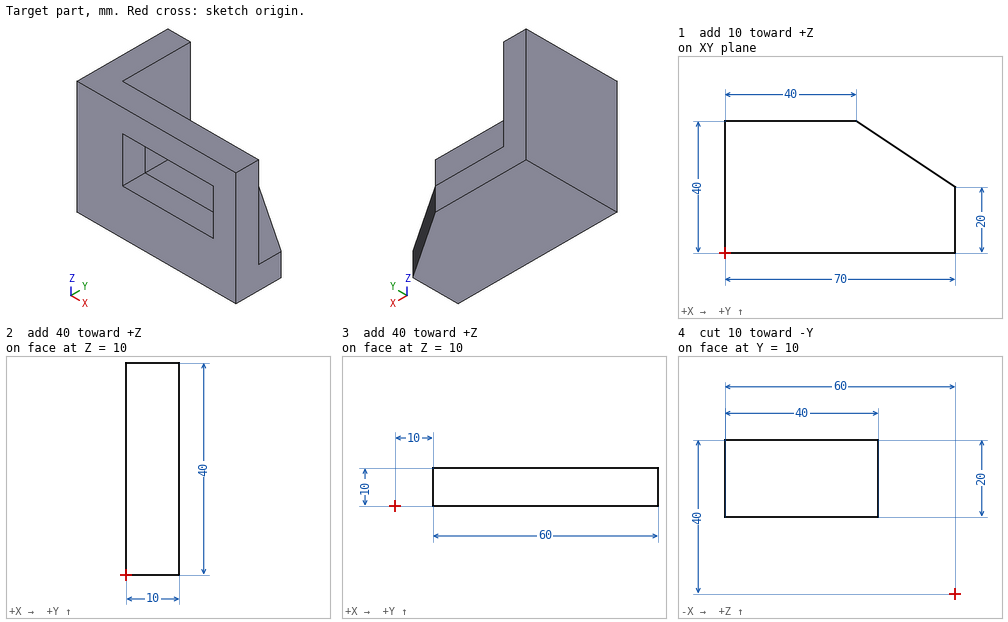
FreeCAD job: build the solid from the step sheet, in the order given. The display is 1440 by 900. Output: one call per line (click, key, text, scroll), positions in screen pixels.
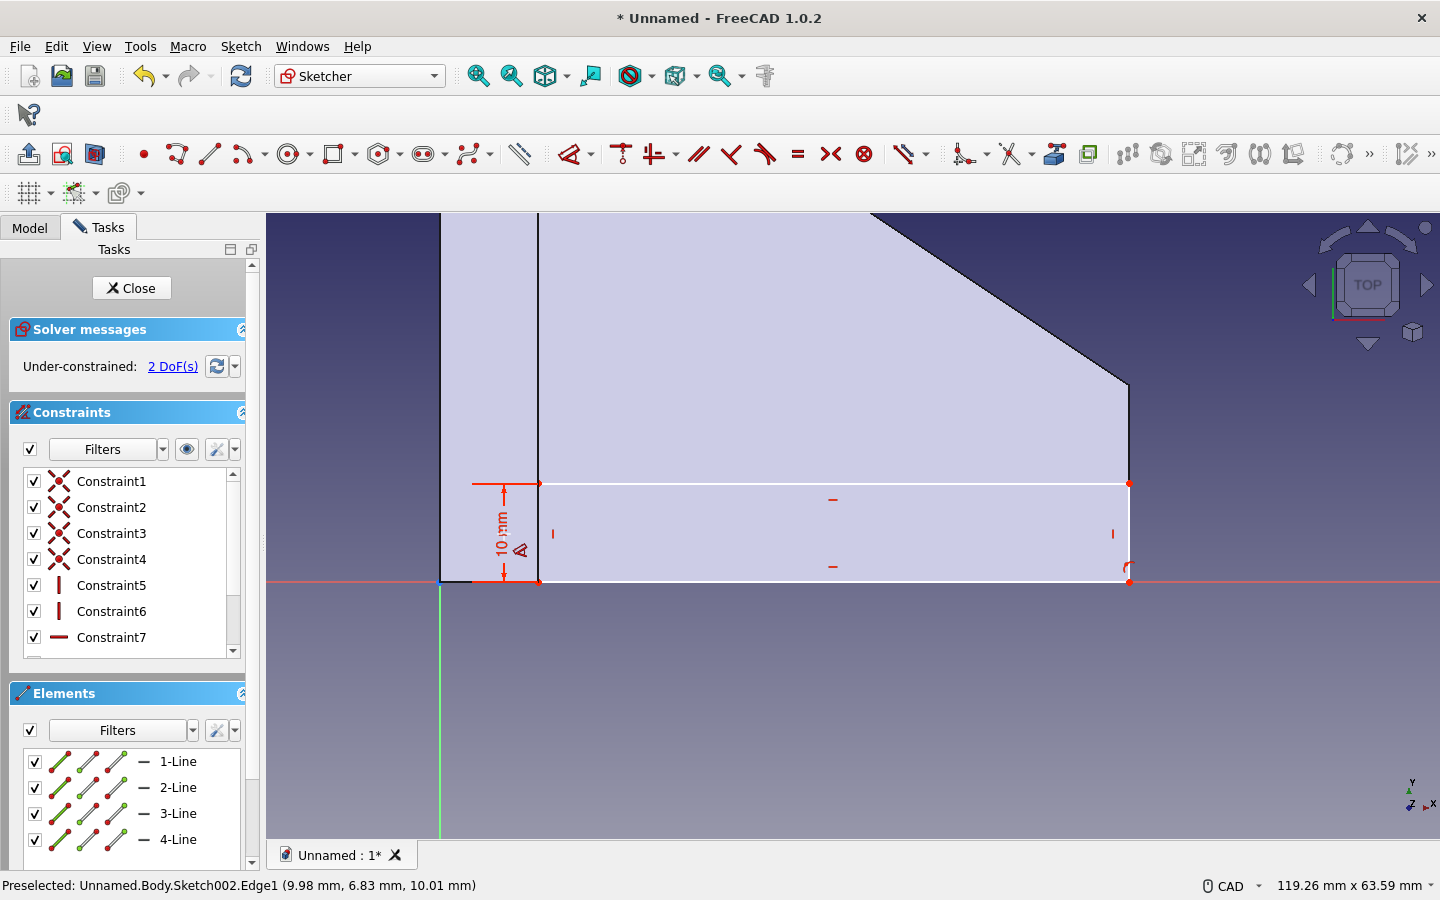
click(715, 582)
click(834, 616)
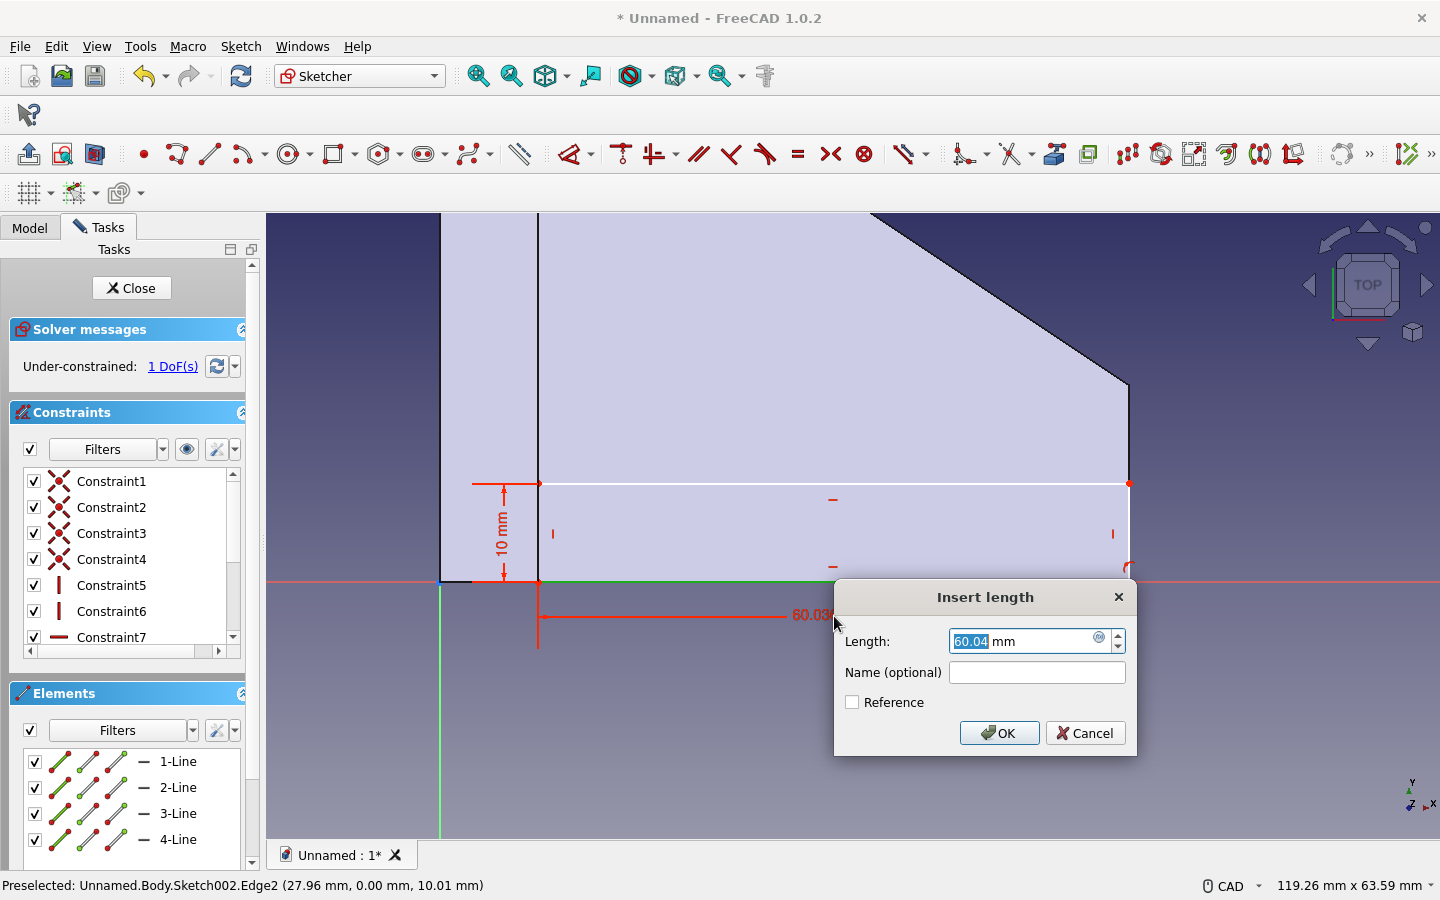
text(60)
key(Return)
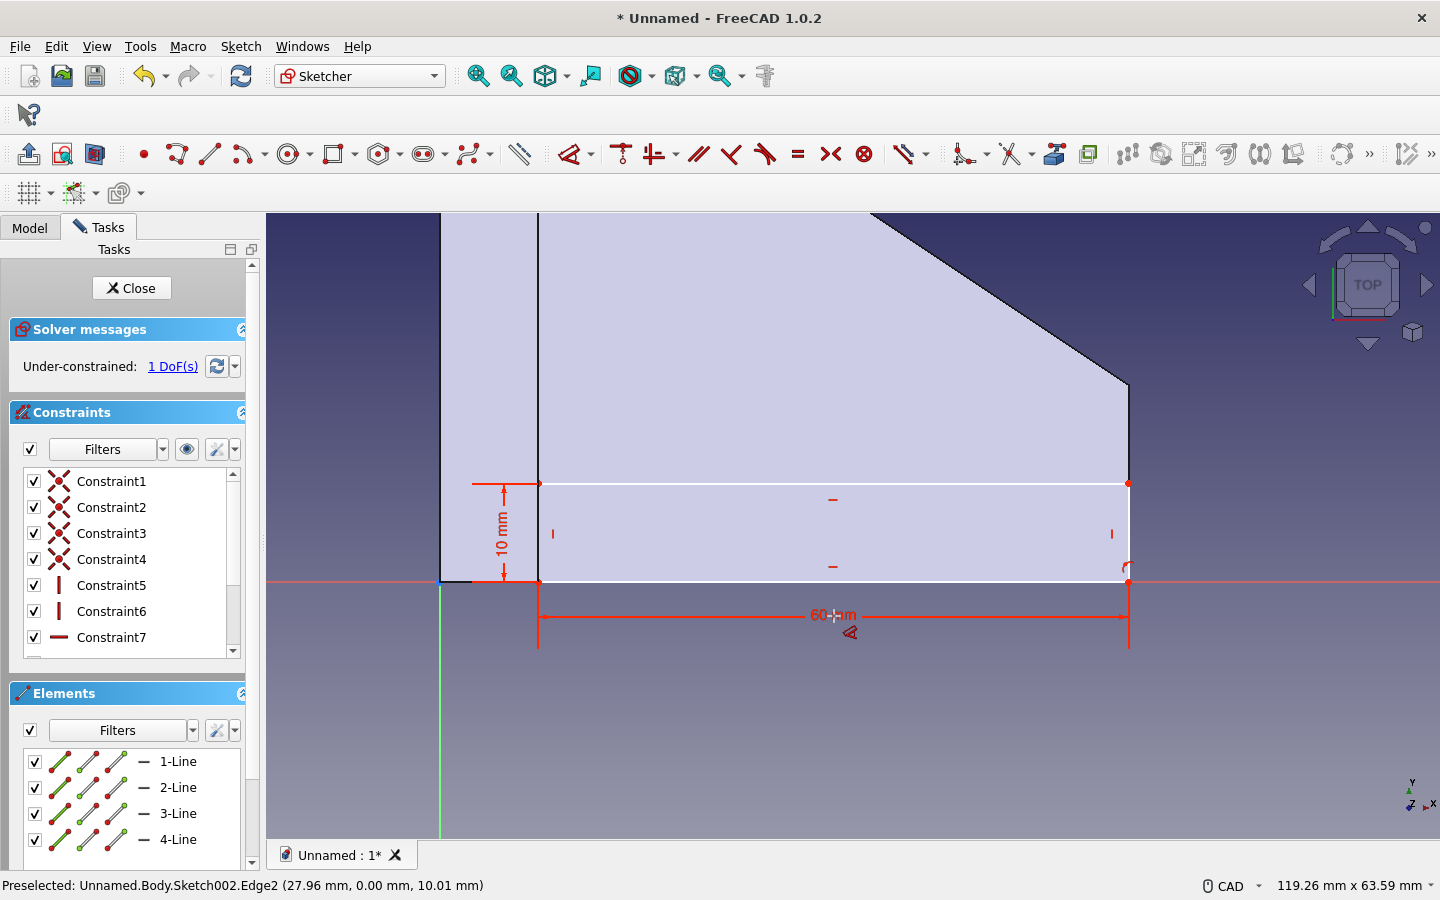
click(538, 484)
click(489, 450)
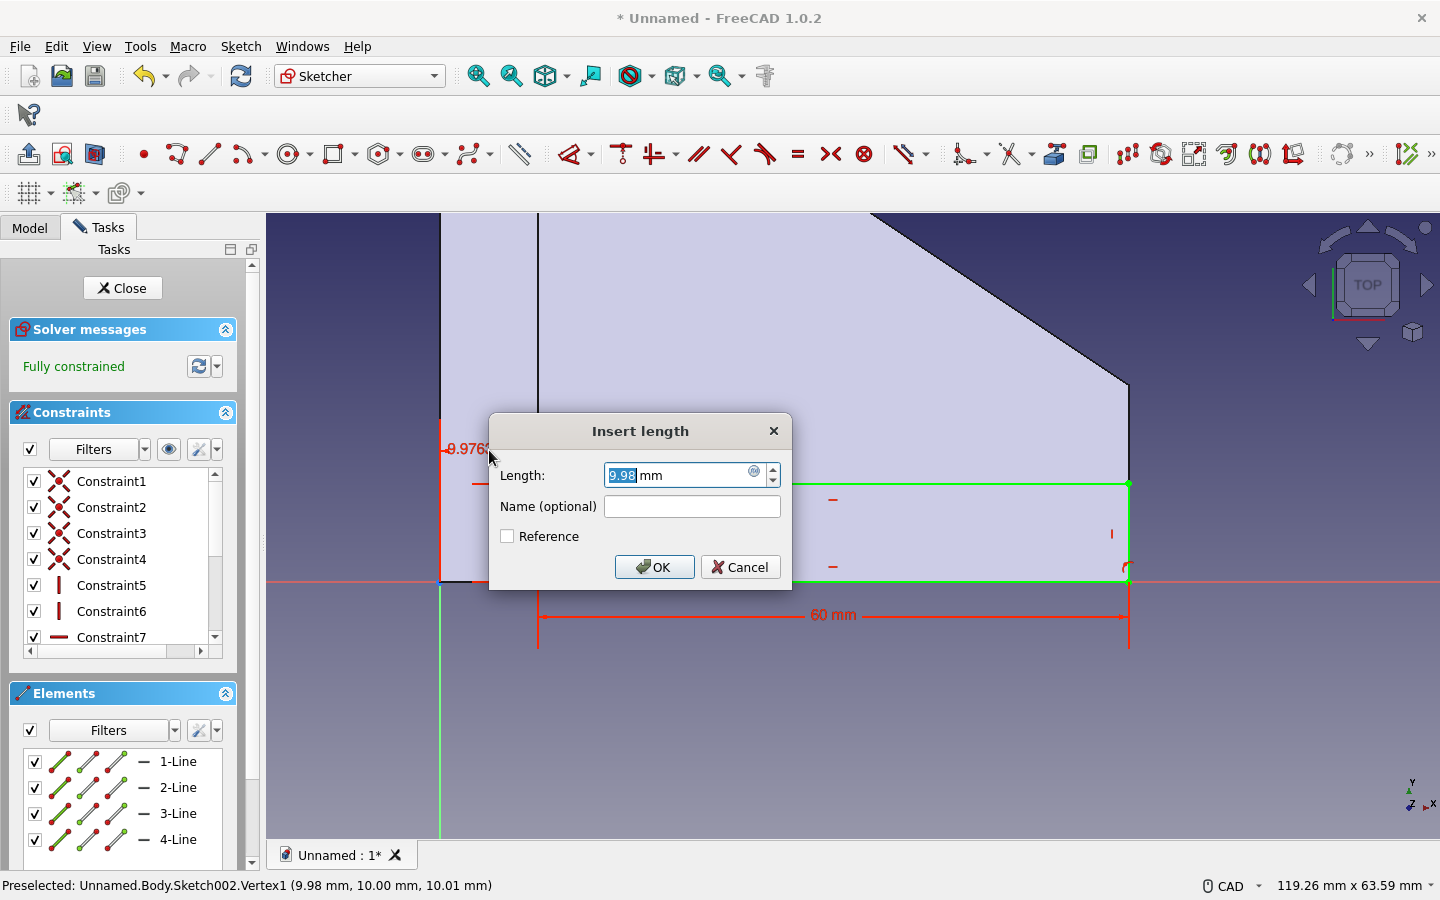
text(10)
key(Return)
key(Escape)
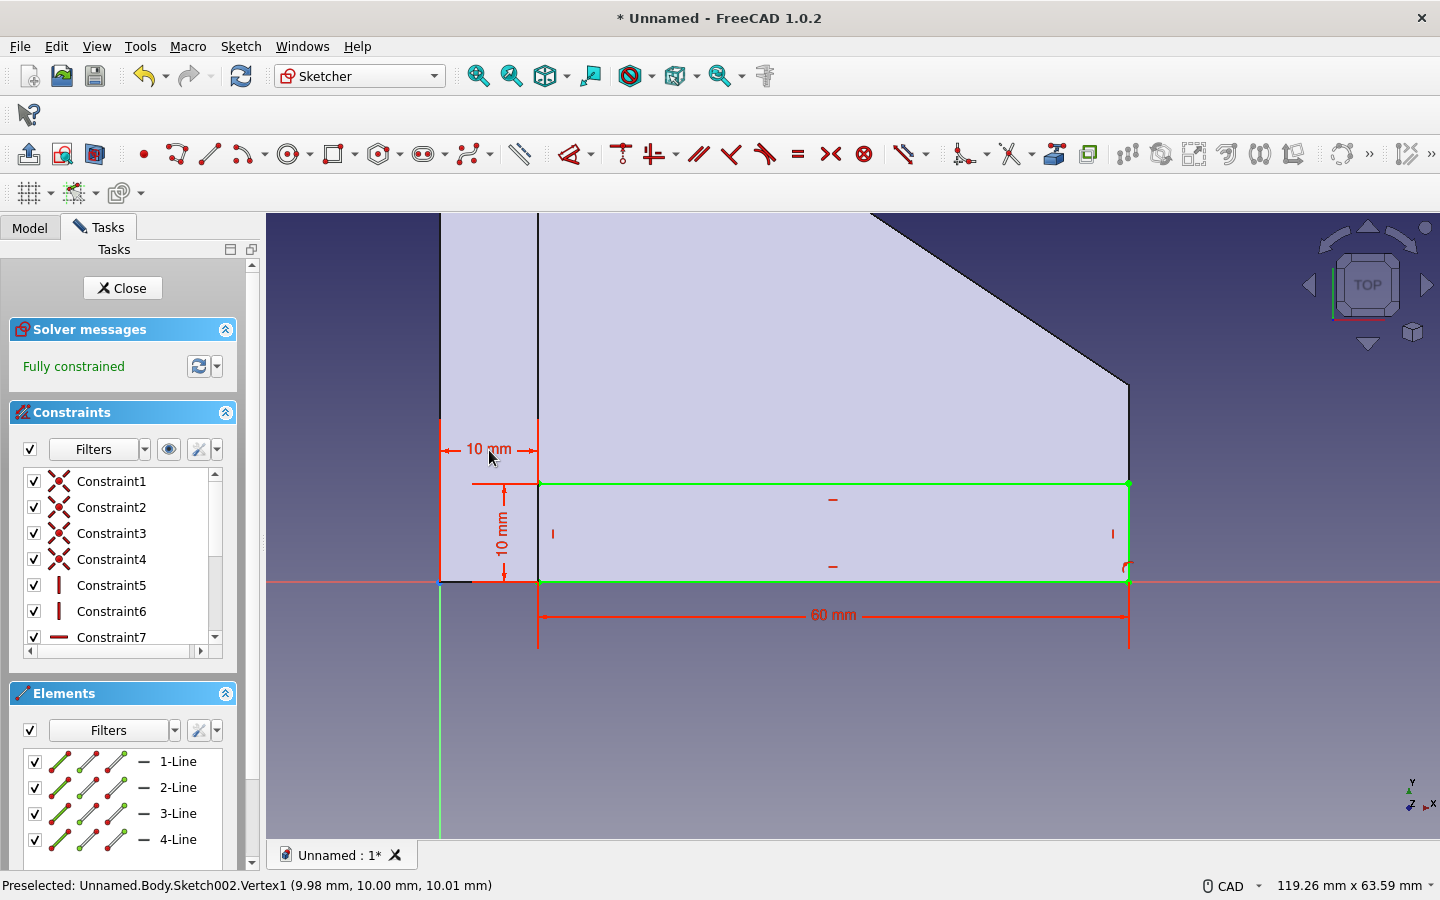
click(123, 288)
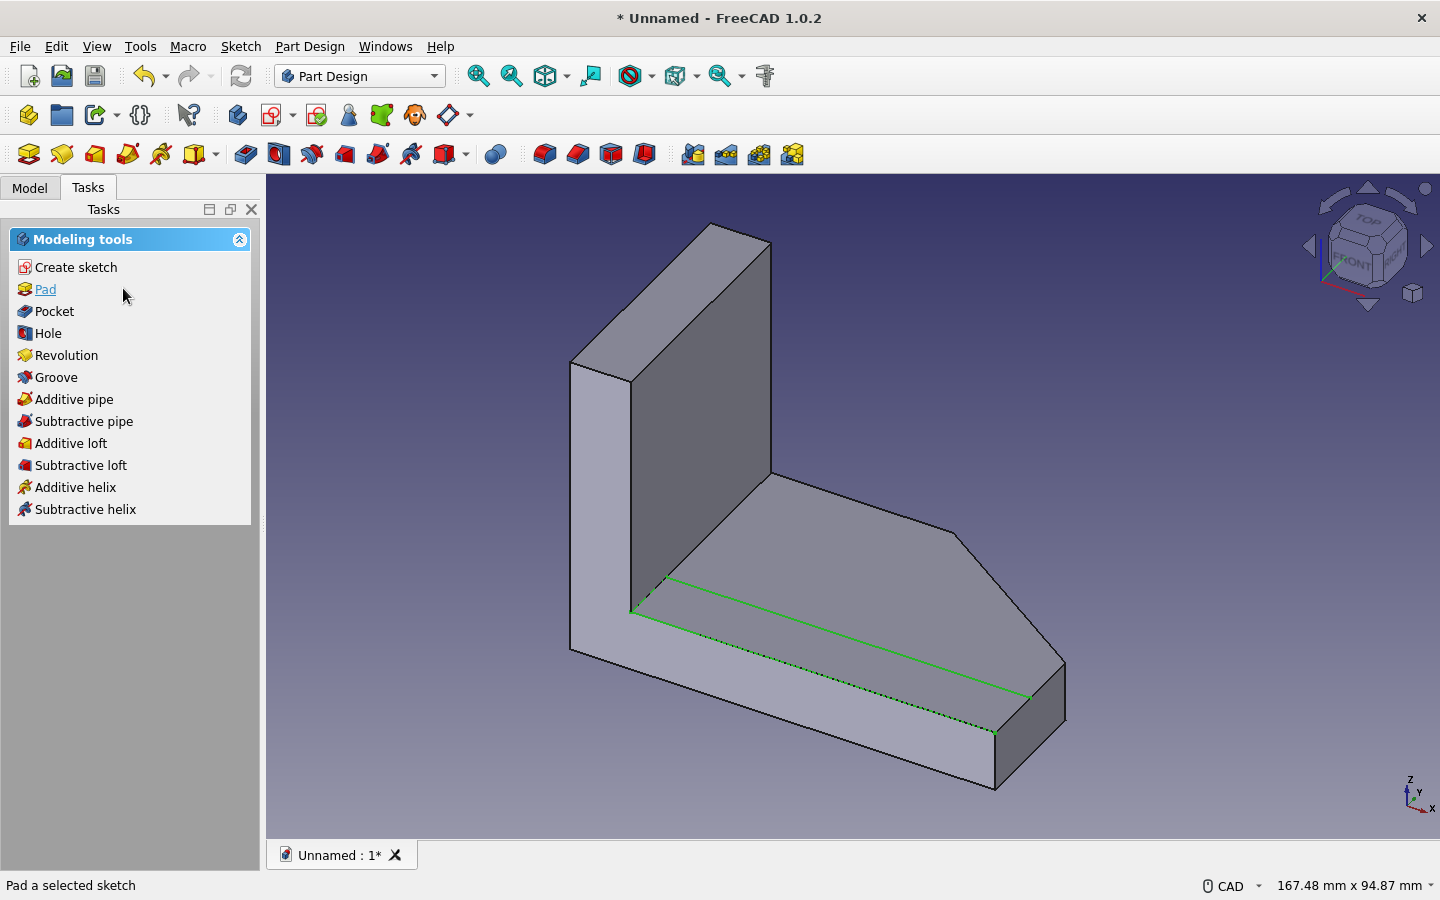
click(29, 154)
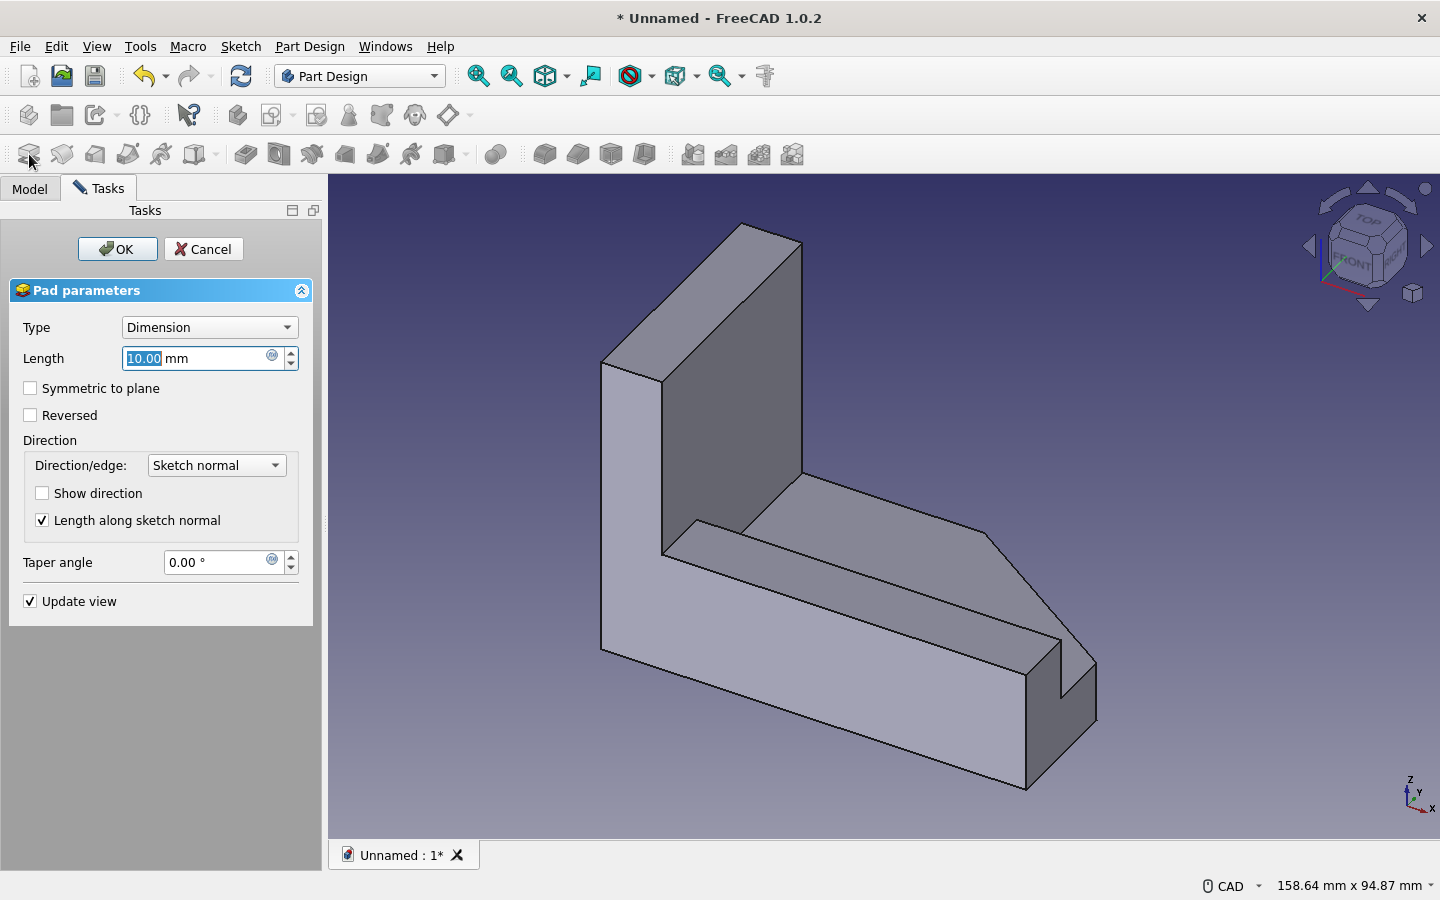
text(40)
key(Tab)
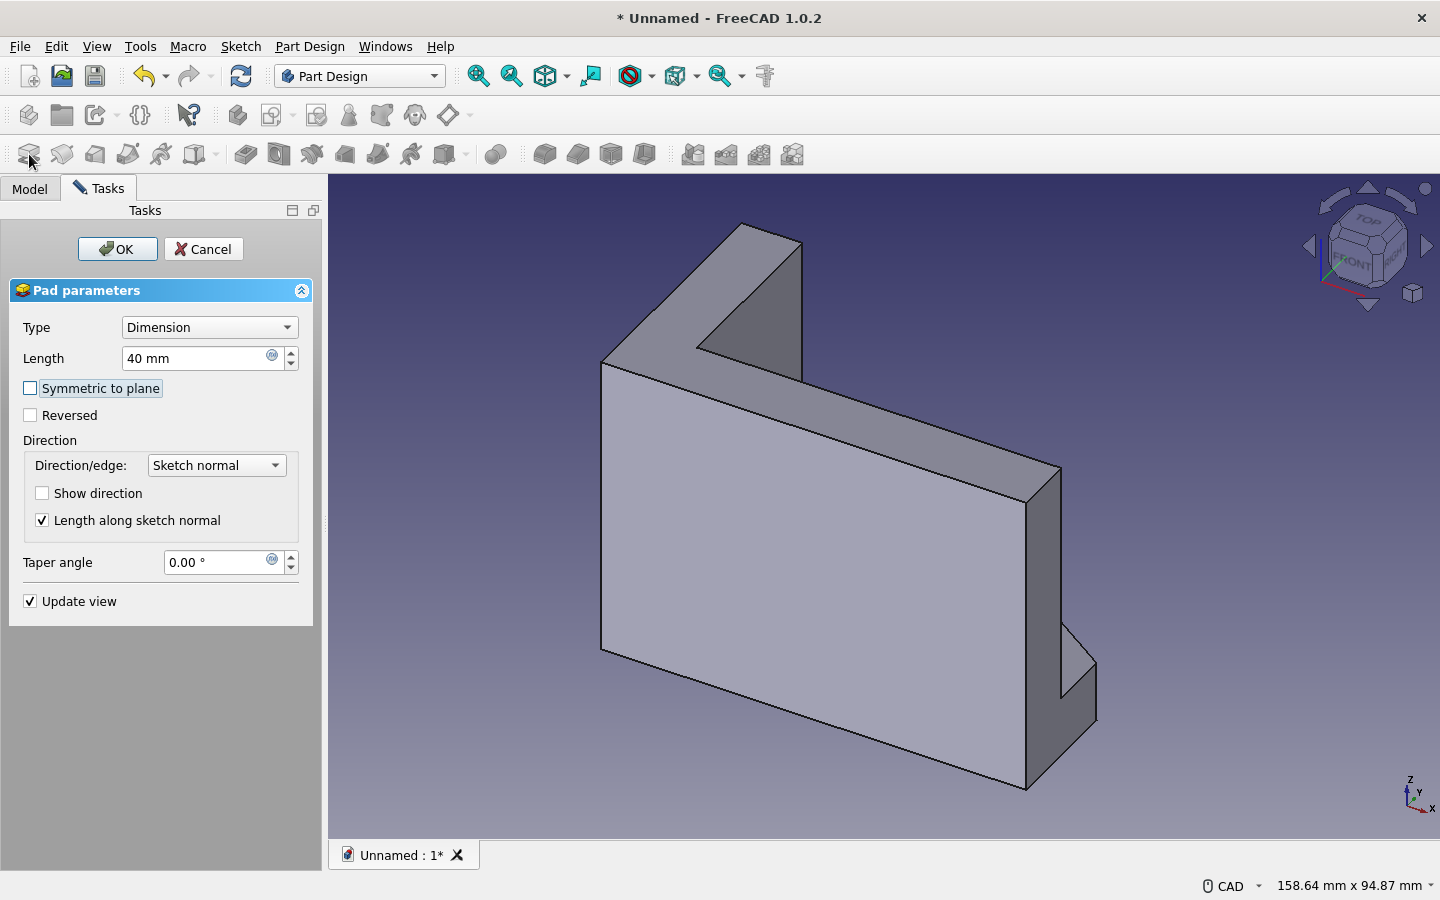
click(118, 249)